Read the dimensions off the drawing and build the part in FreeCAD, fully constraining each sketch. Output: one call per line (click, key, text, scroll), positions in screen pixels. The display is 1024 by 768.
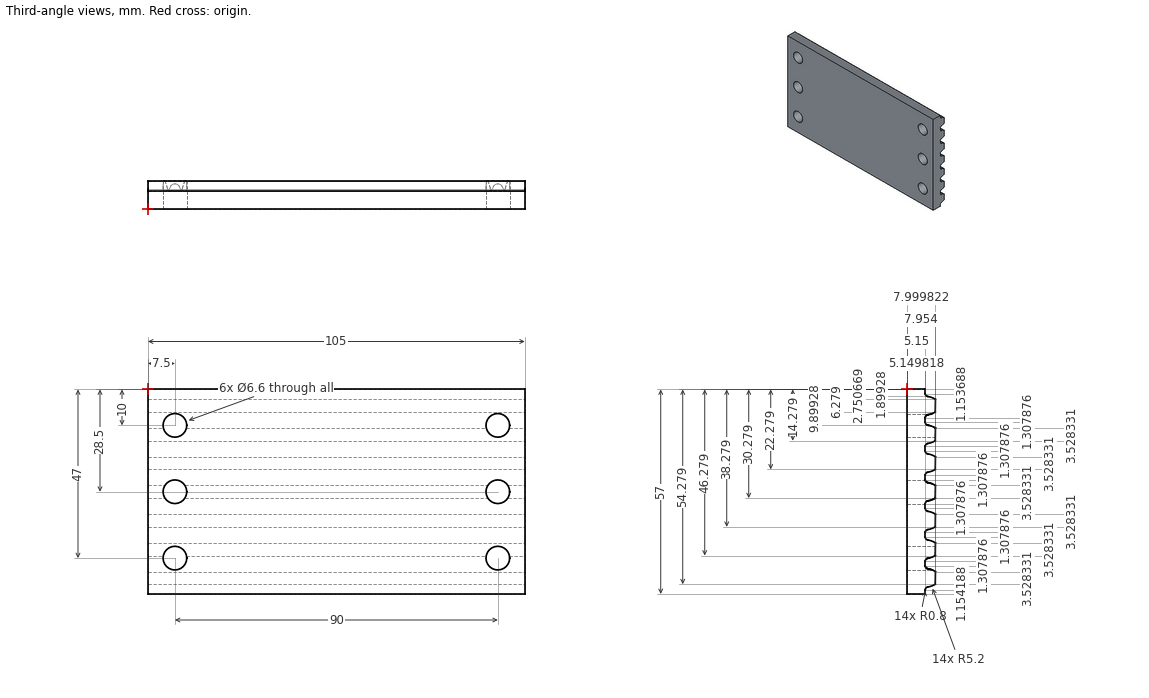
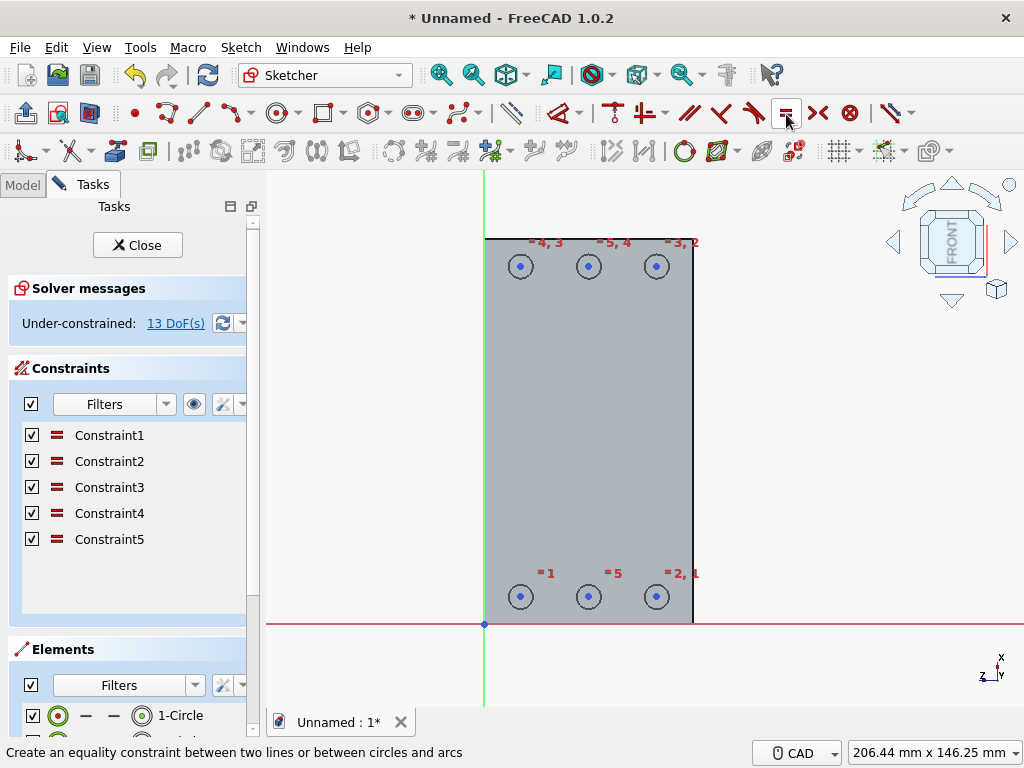
click(521, 597)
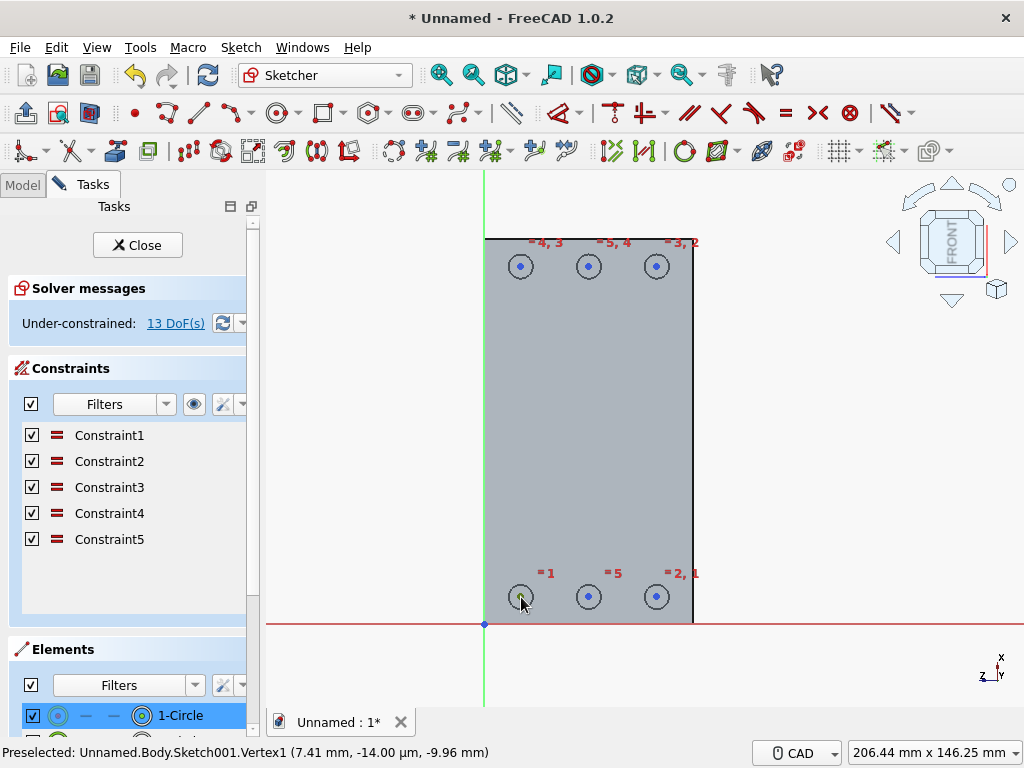
click(657, 597)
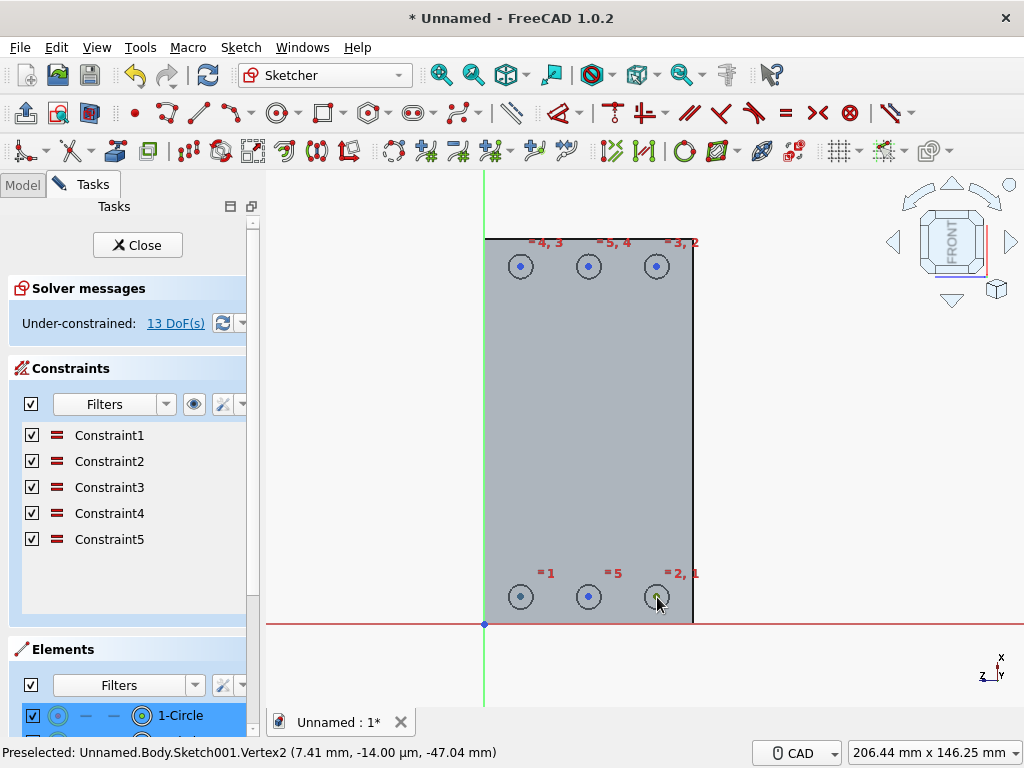
click(668, 114)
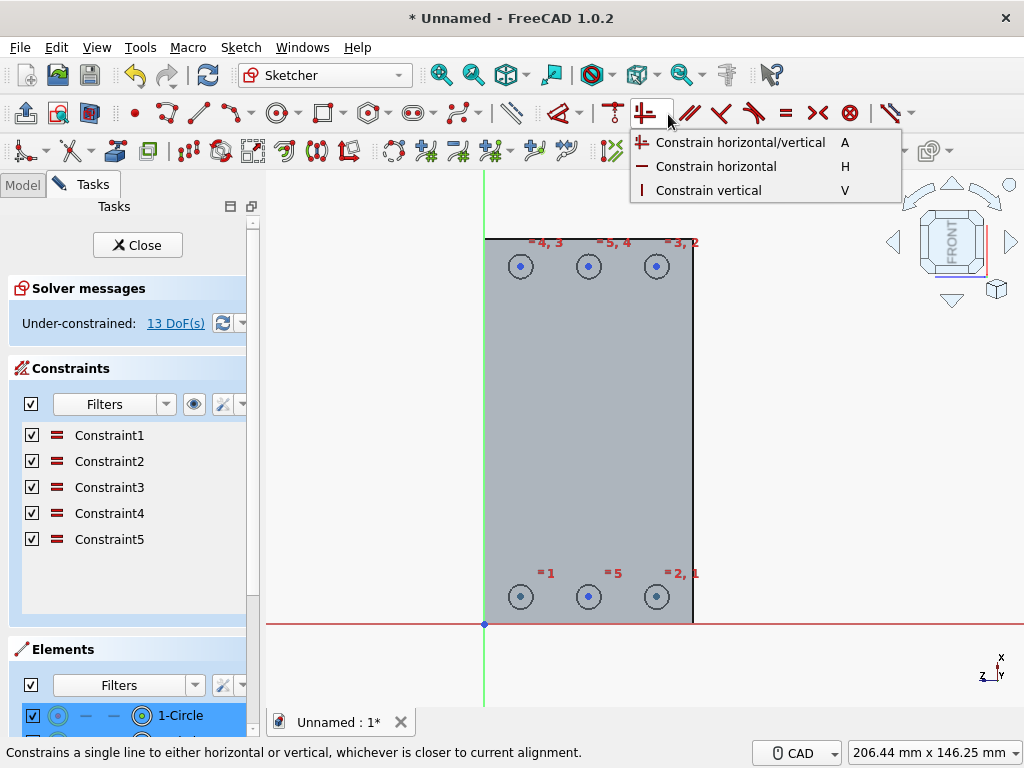
click(766, 166)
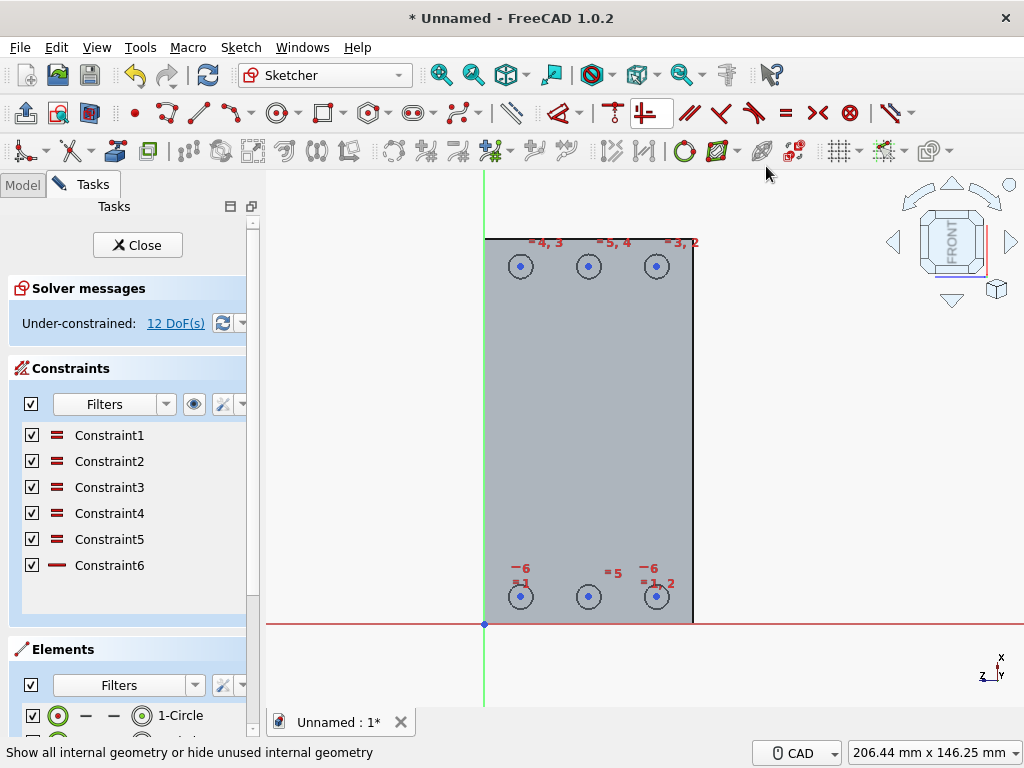
click(657, 597)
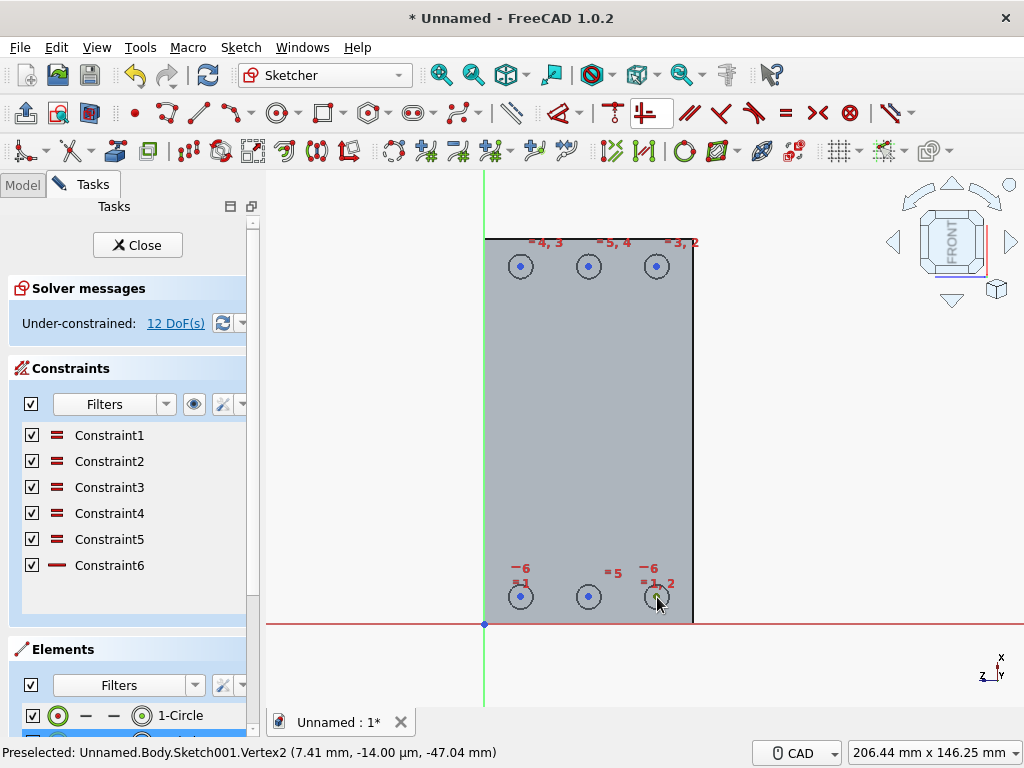
click(657, 267)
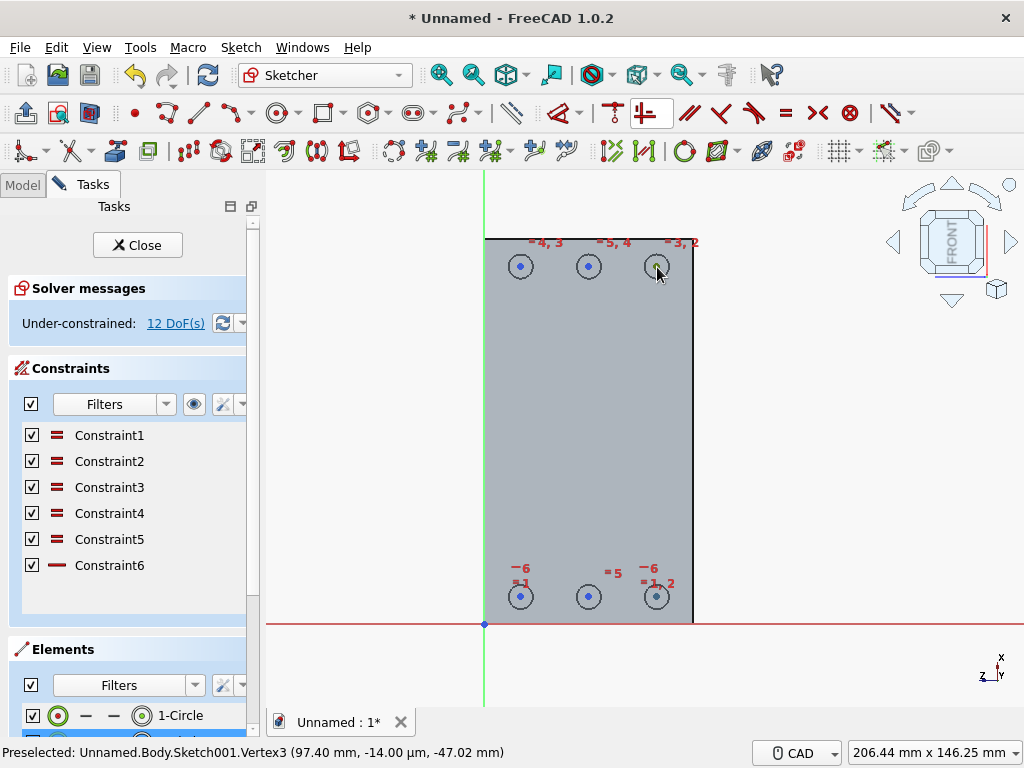
click(668, 114)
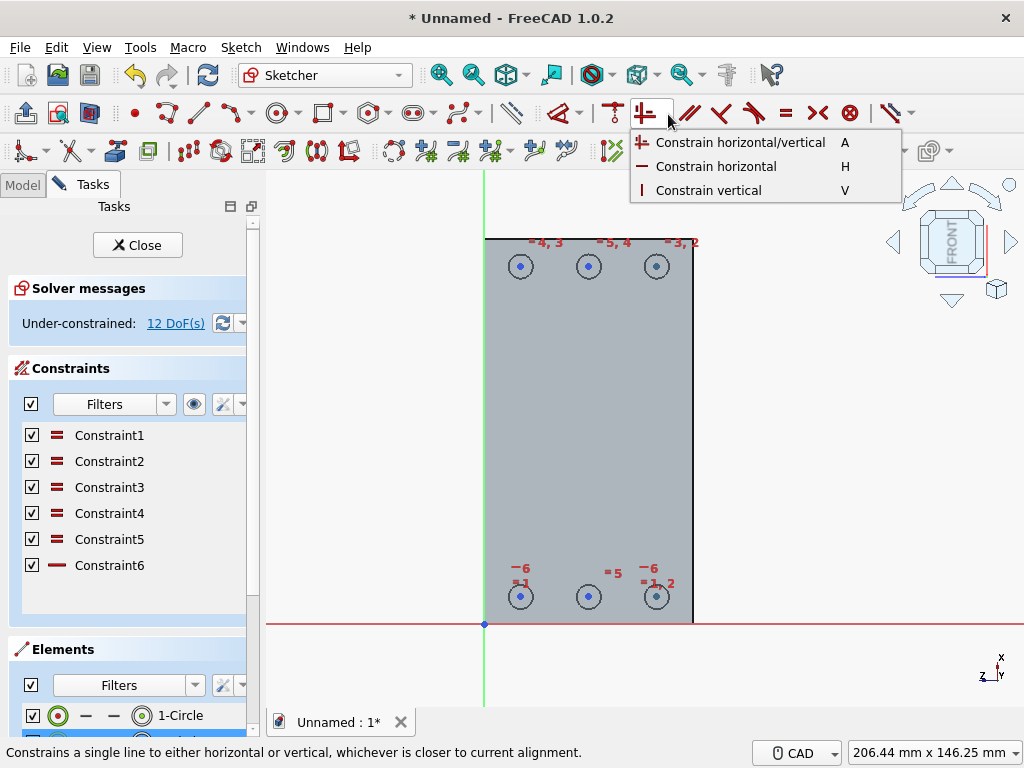
click(766, 190)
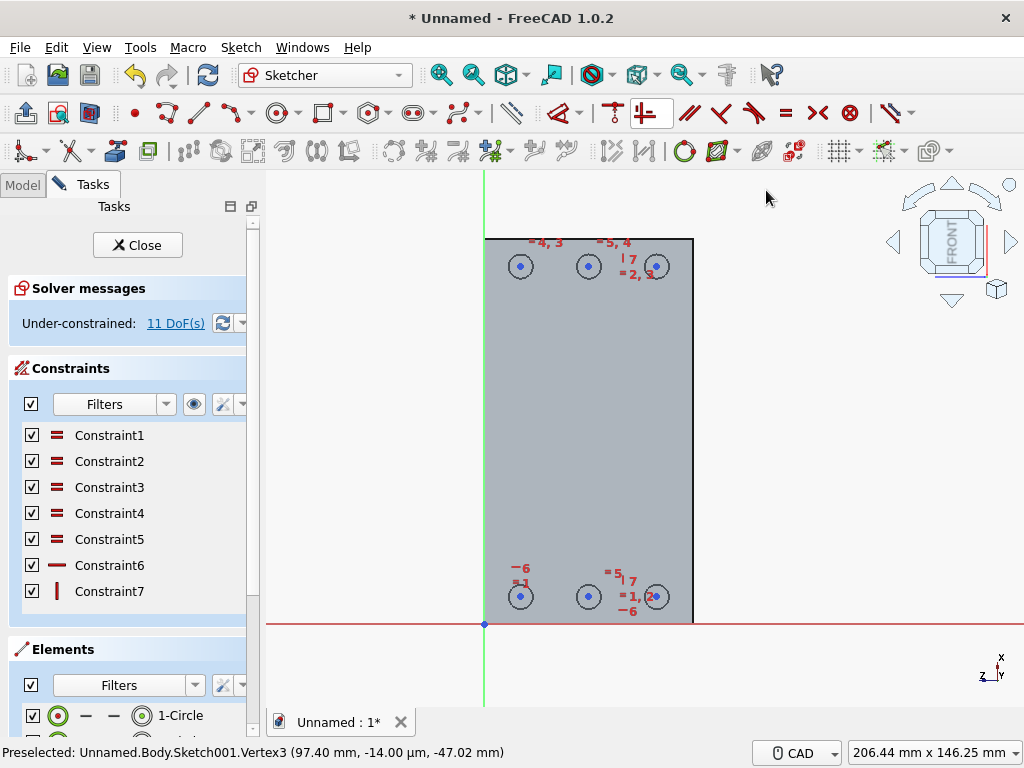
click(521, 597)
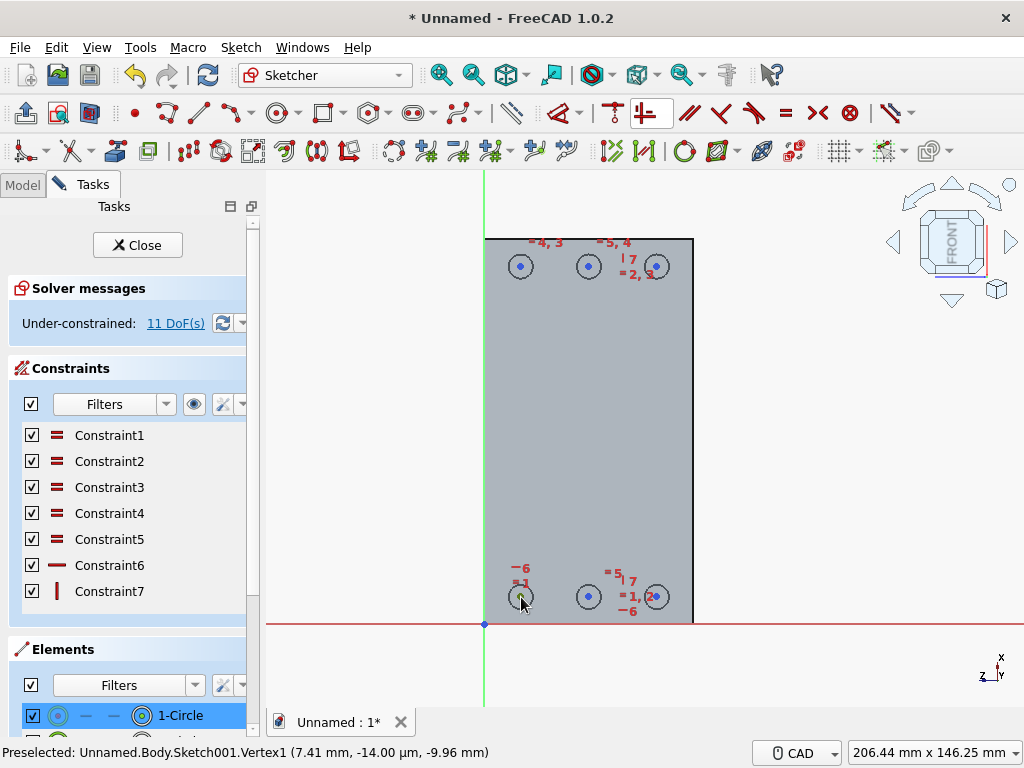
click(521, 267)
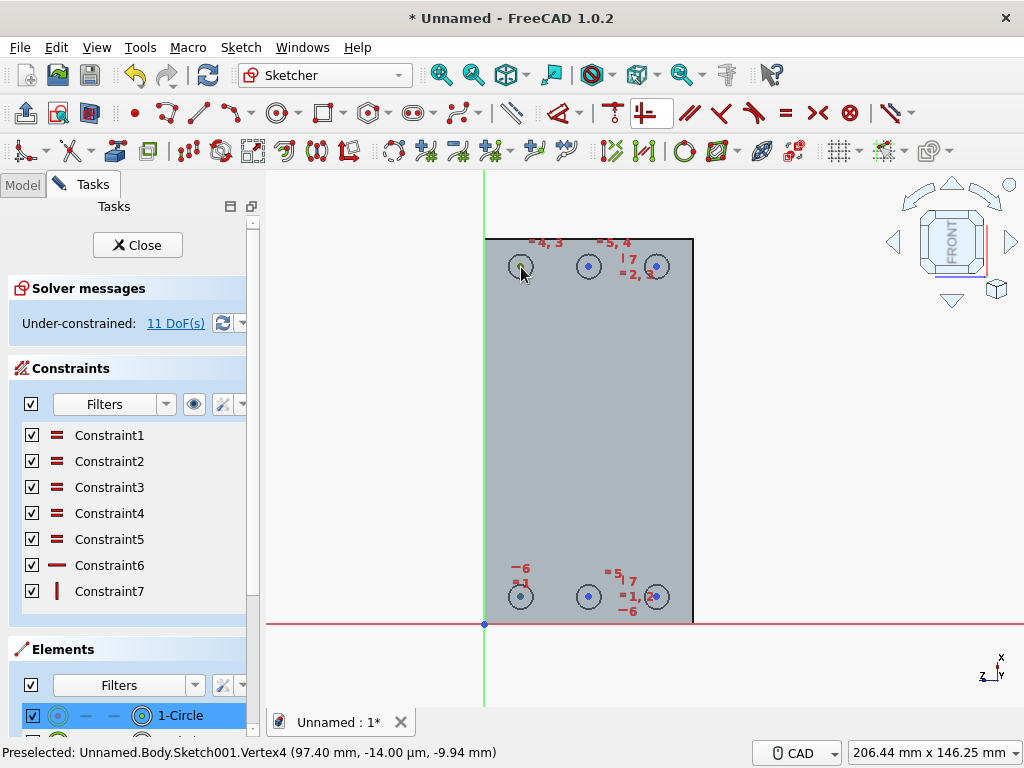
click(668, 114)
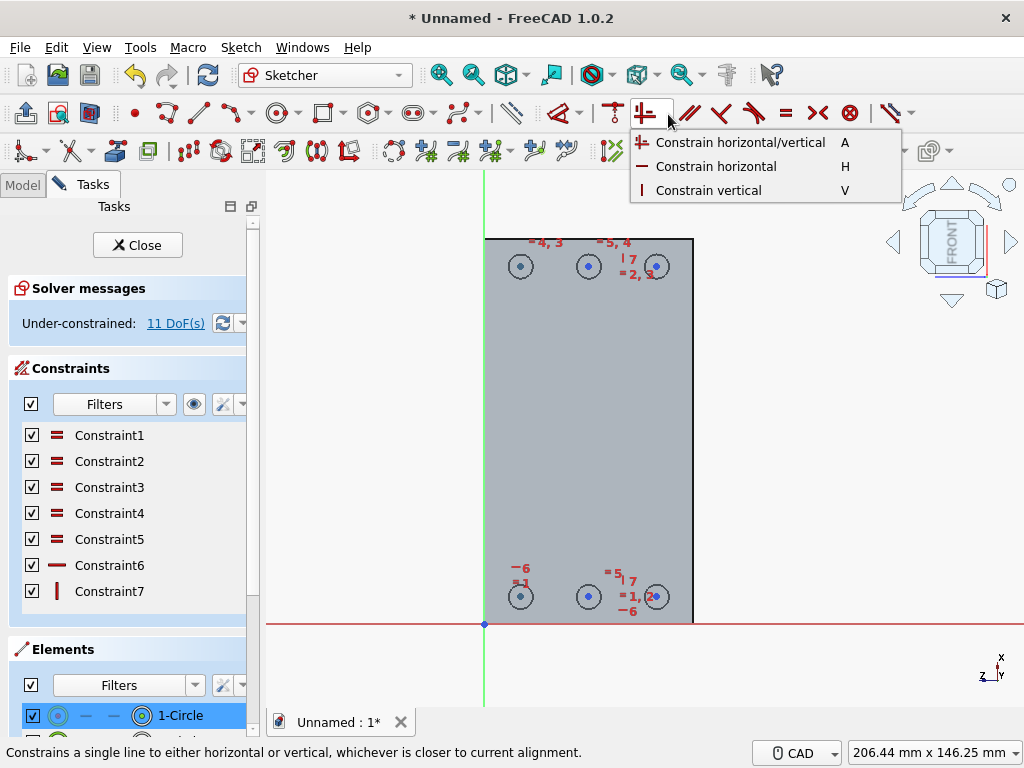
click(766, 190)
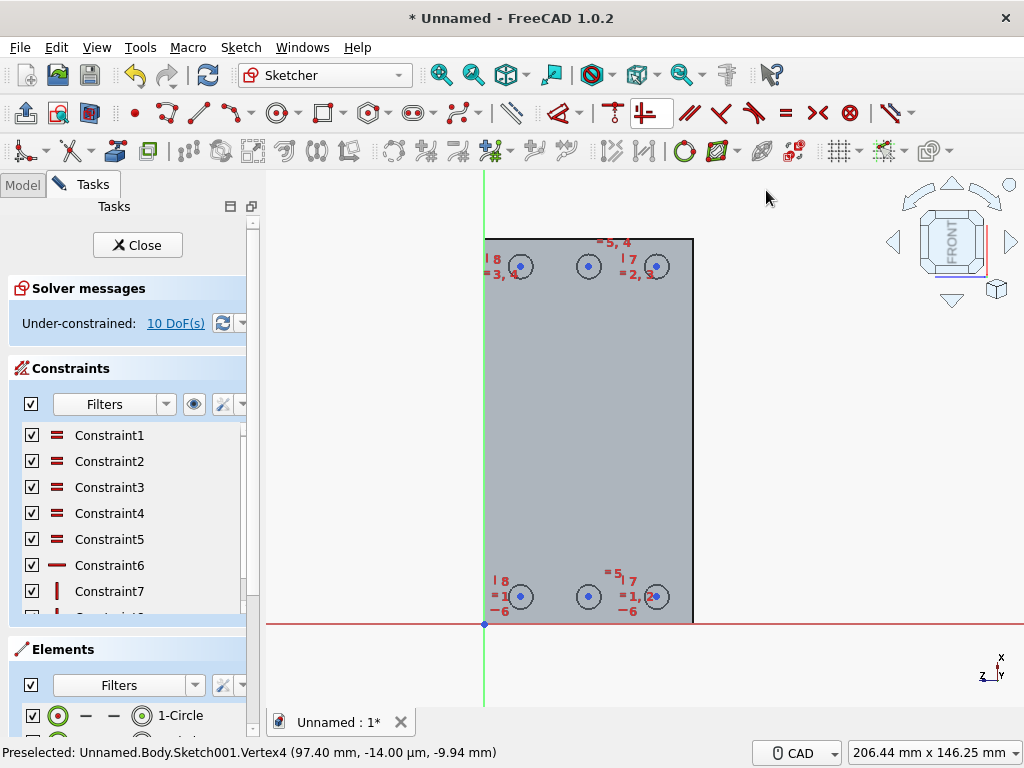
click(657, 267)